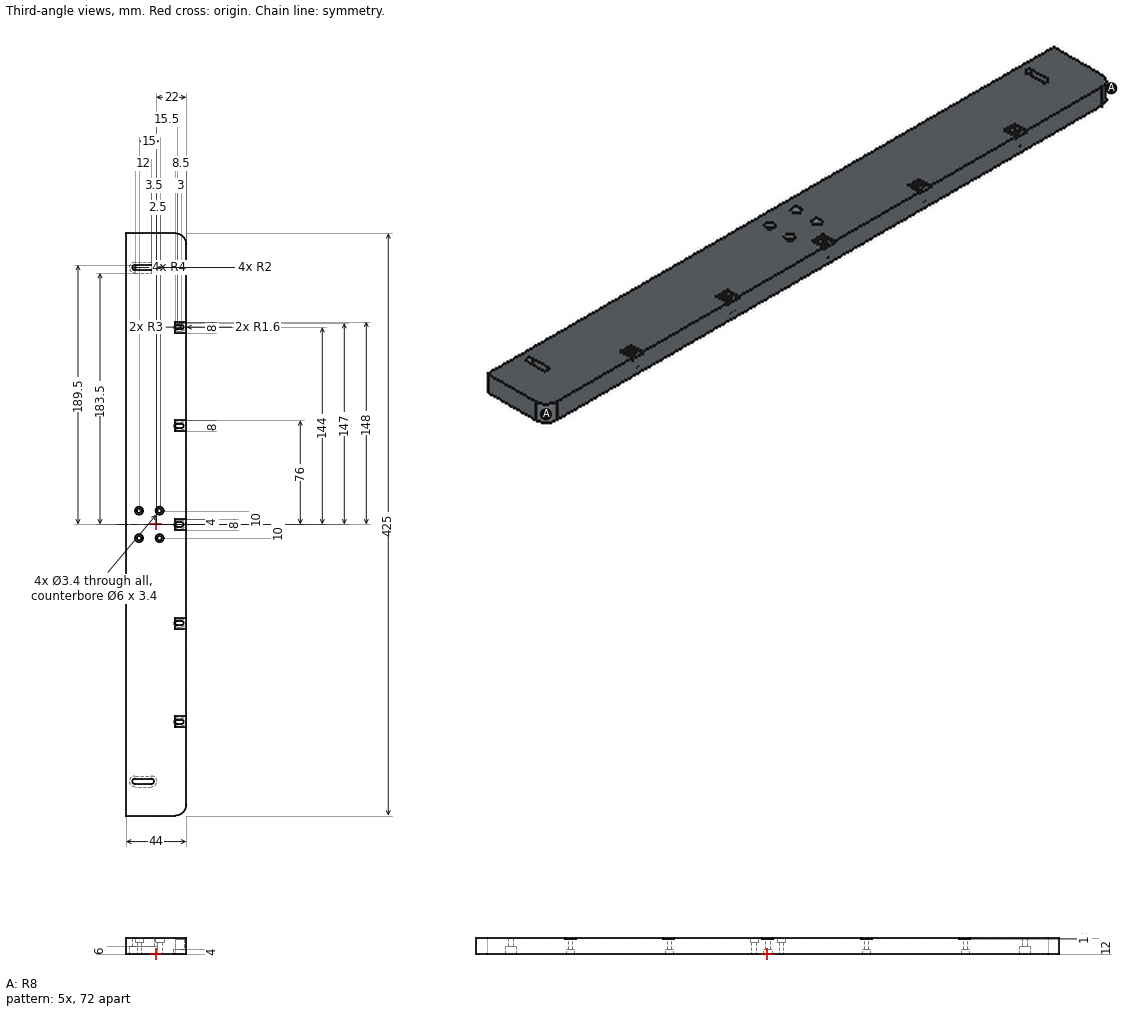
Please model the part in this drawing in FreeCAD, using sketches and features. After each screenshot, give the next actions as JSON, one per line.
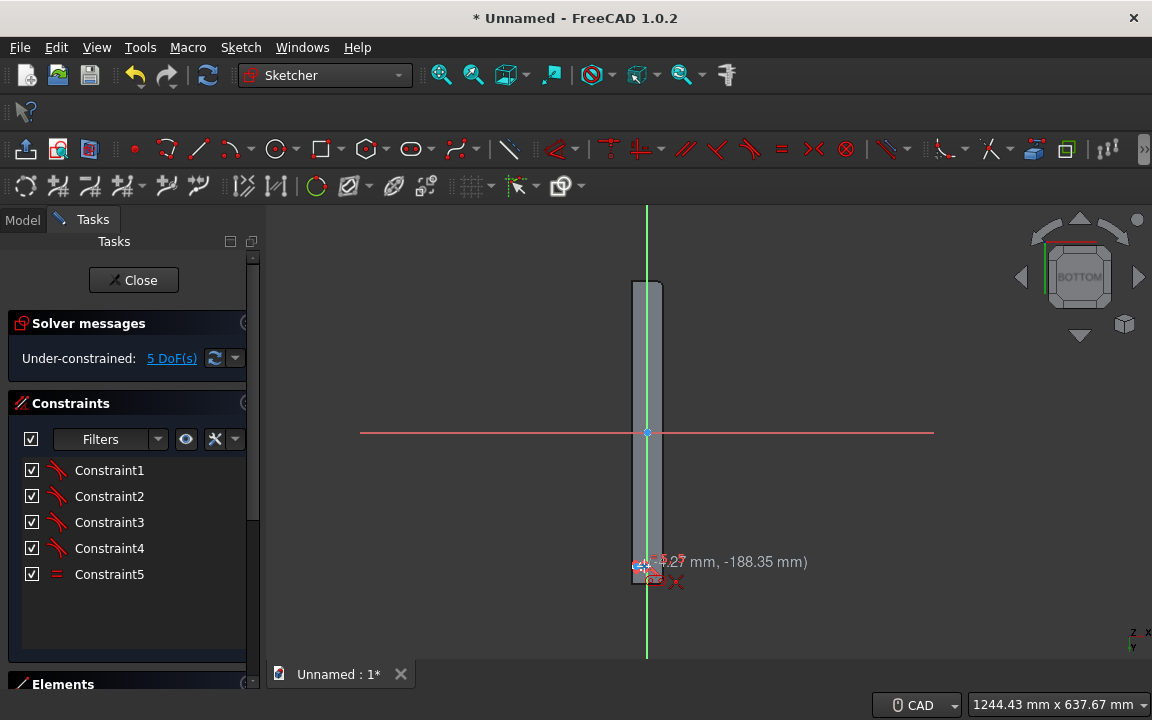
{"action": "scroll", "coordinate": [636, 299], "scroll_direction": "up", "scroll_amount": 11}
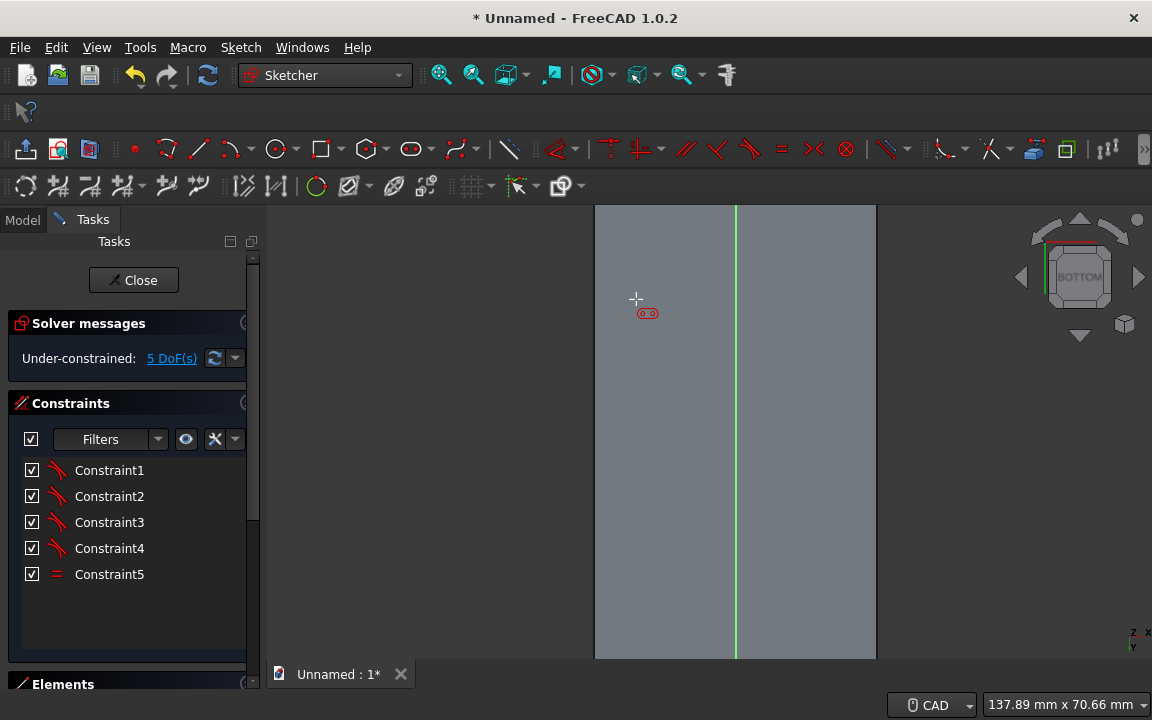
{"action": "scroll", "coordinate": [636, 298], "scroll_direction": "down", "scroll_amount": 11}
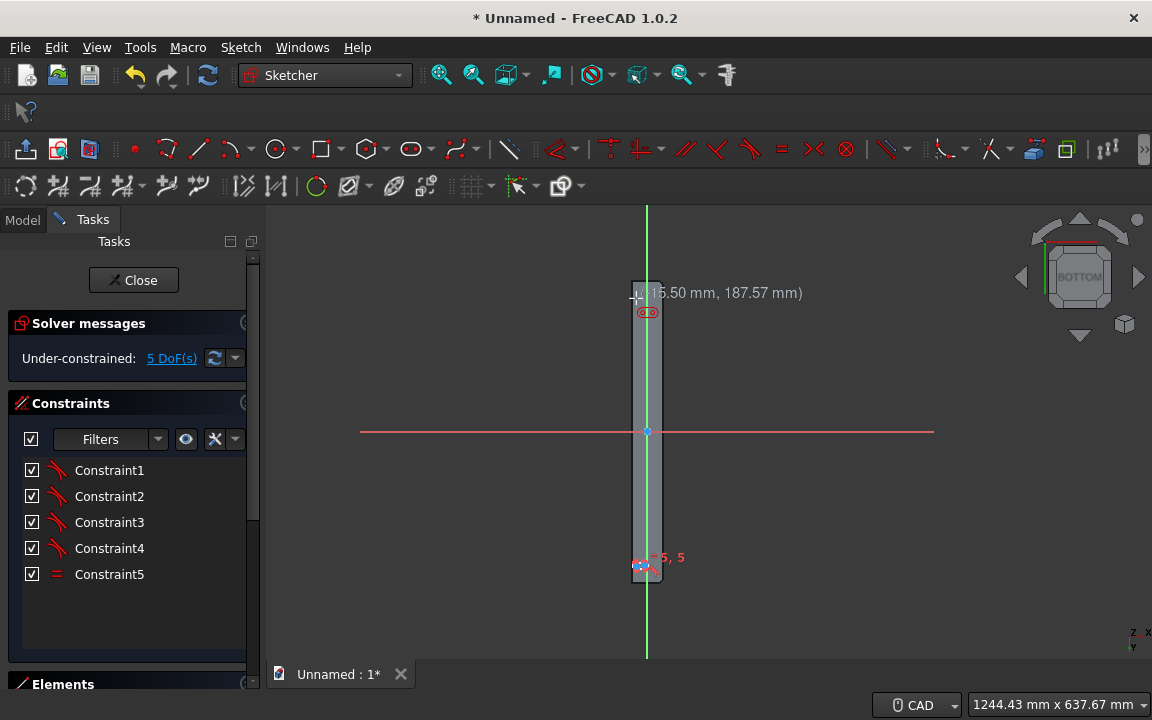
{"action": "scroll", "coordinate": [636, 298], "scroll_direction": "up", "scroll_amount": 2}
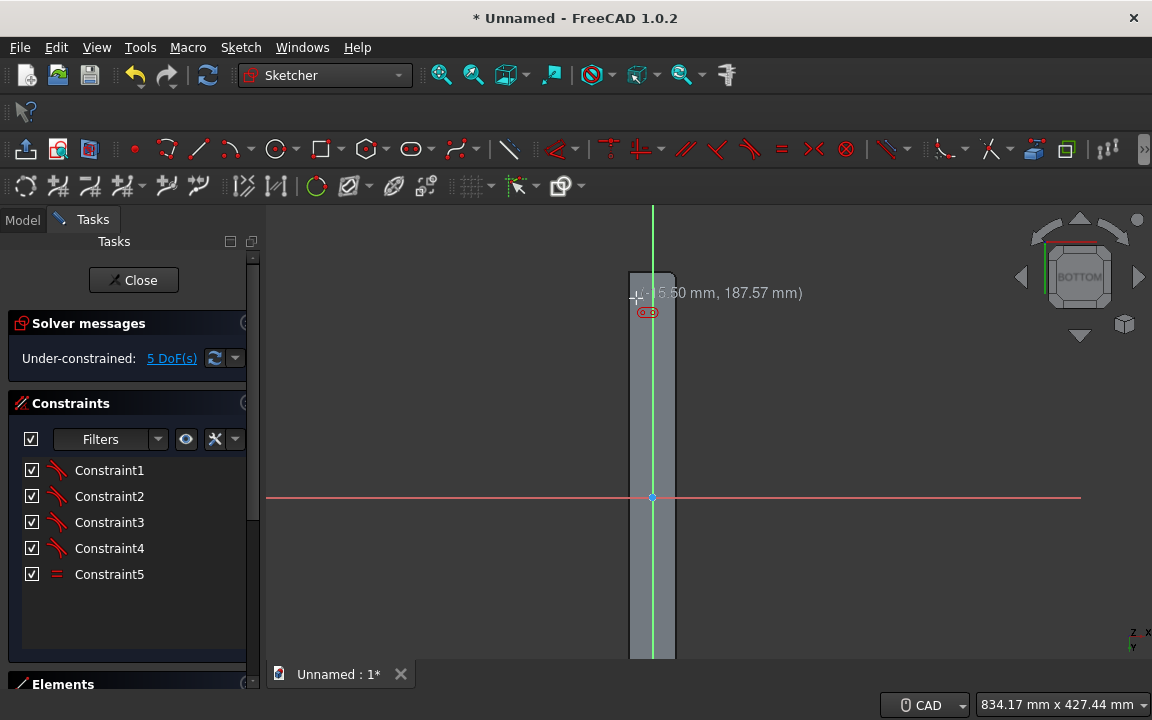
{"action": "left_click", "coordinate": [636, 298]}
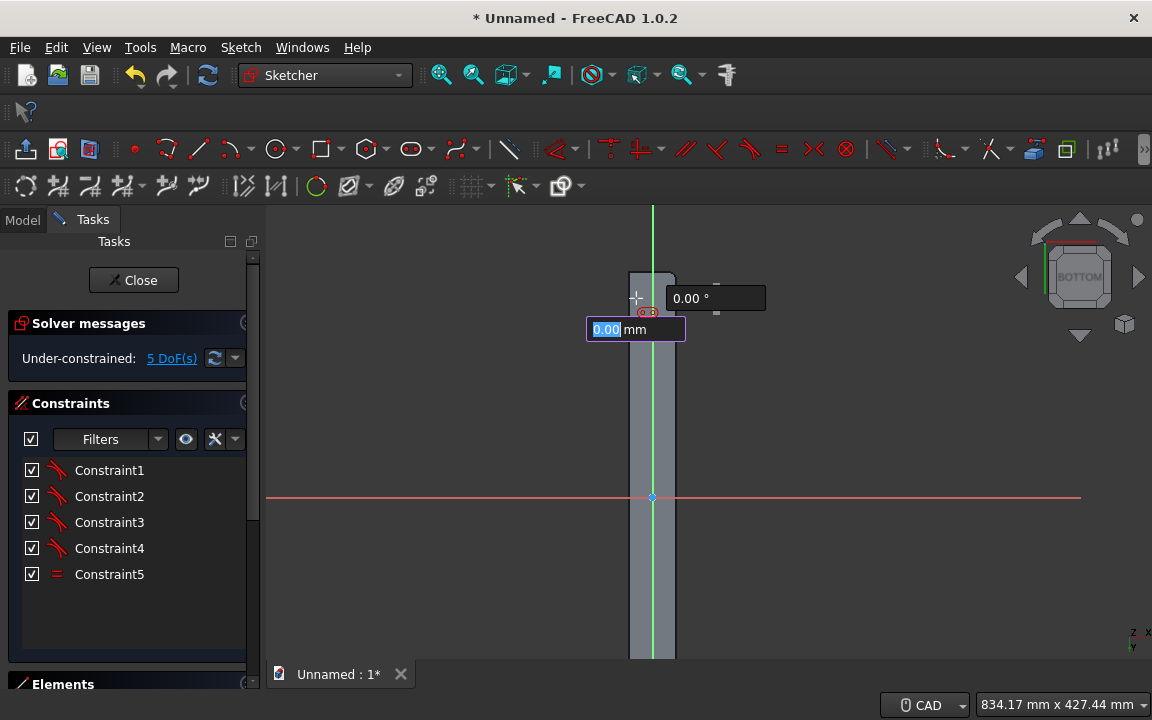
{"action": "scroll", "coordinate": [649, 298], "scroll_direction": "up", "scroll_amount": 8}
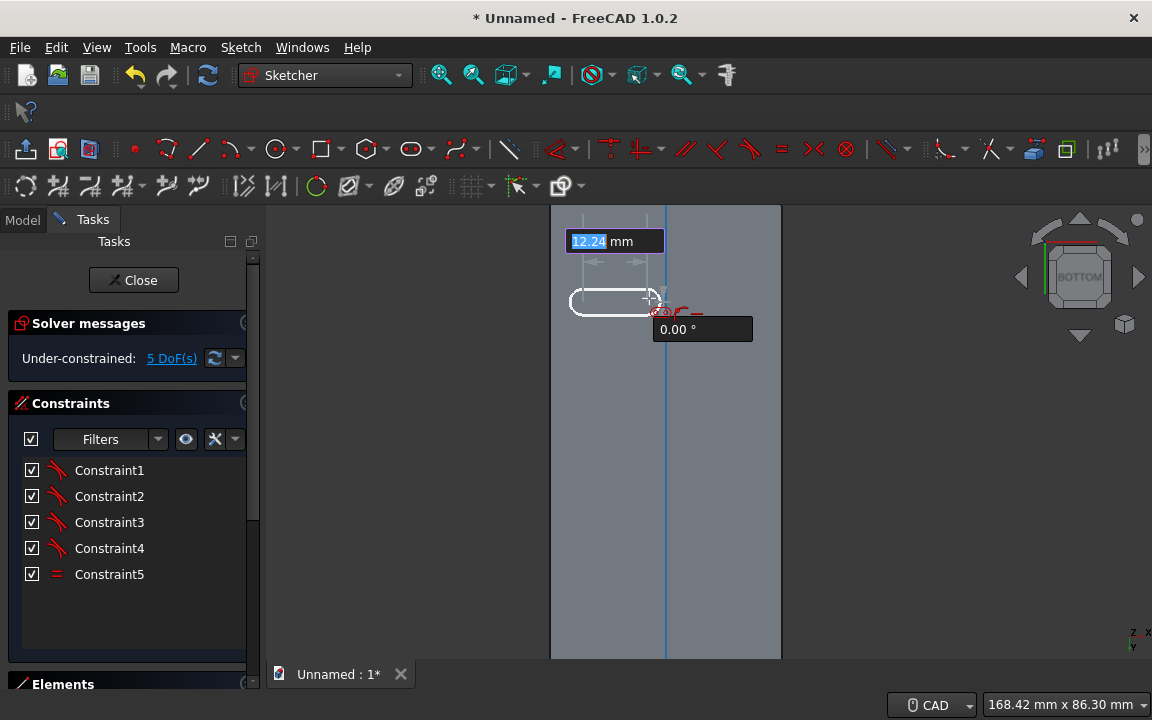
{"action": "left_click", "coordinate": [648, 297]}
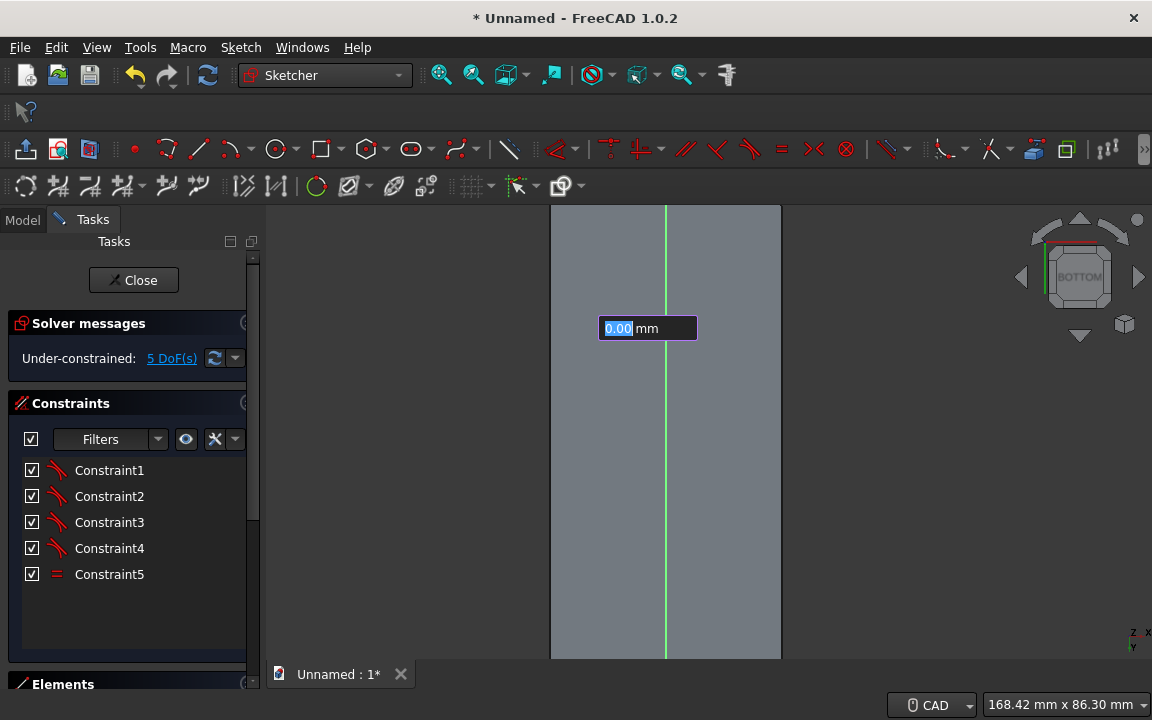
{"action": "left_click", "coordinate": [616, 320]}
{"action": "key", "text": "Escape"}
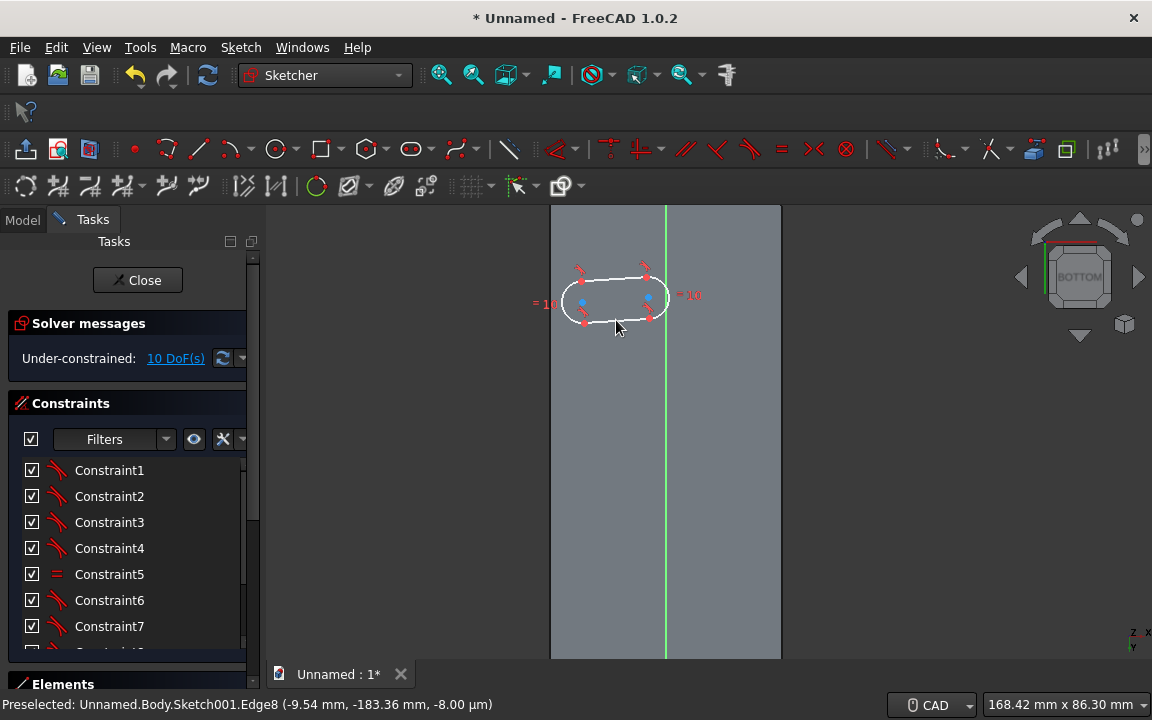
{"action": "scroll", "coordinate": [644, 298], "scroll_direction": "down", "scroll_amount": 10}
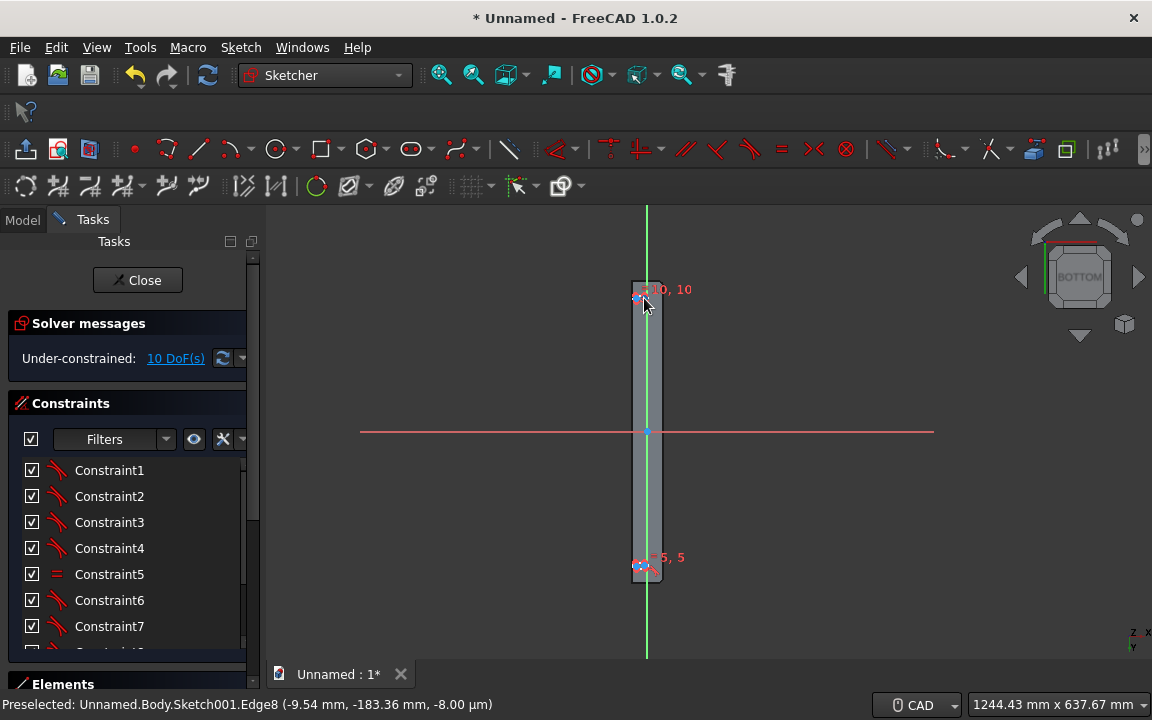
{"action": "scroll", "coordinate": [639, 563], "scroll_direction": "up", "scroll_amount": 9}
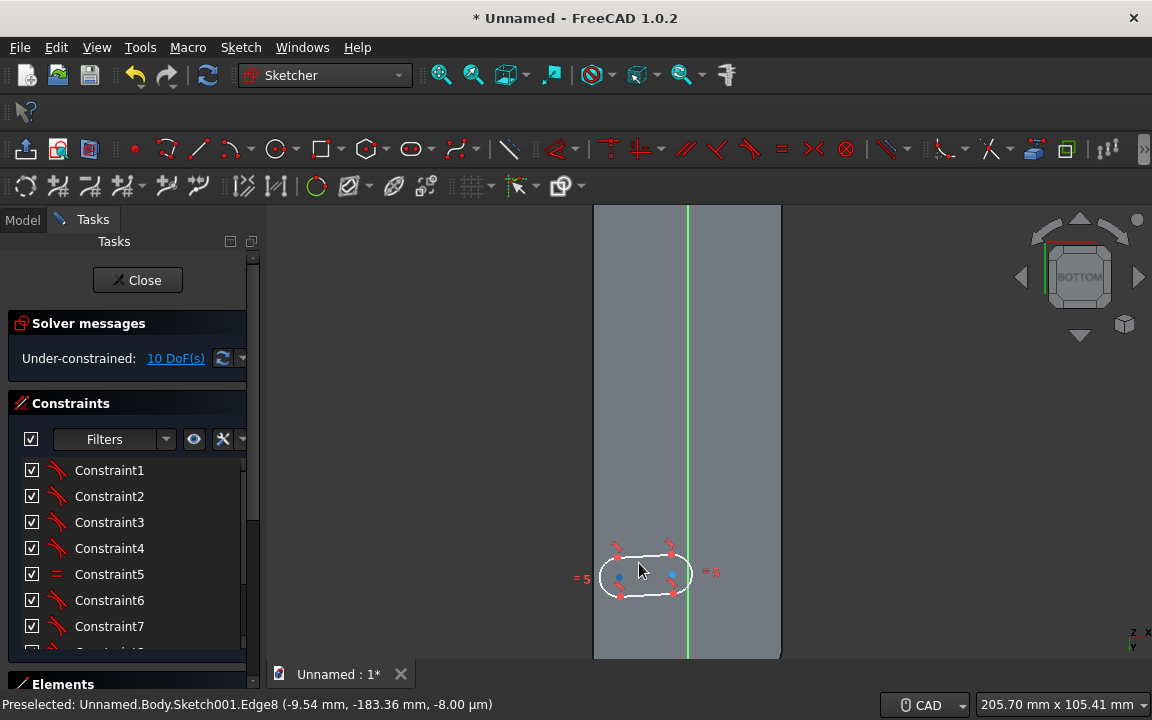
{"action": "left_click", "coordinate": [634, 557]}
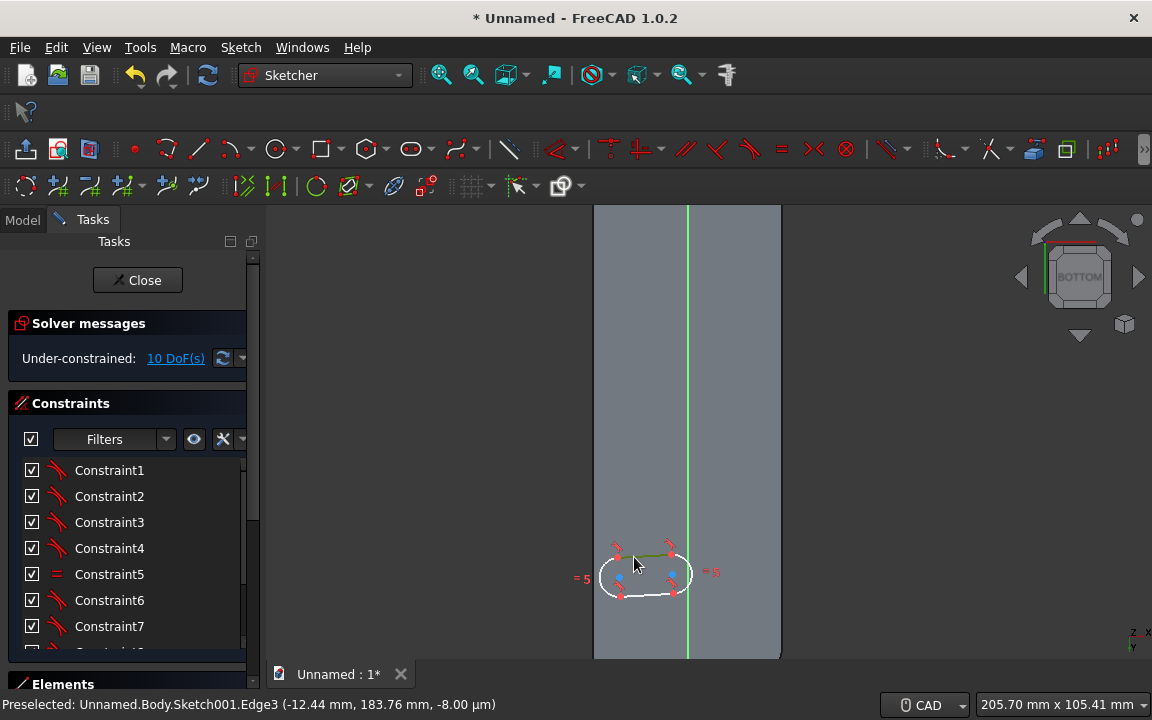
{"action": "left_click", "coordinate": [664, 150]}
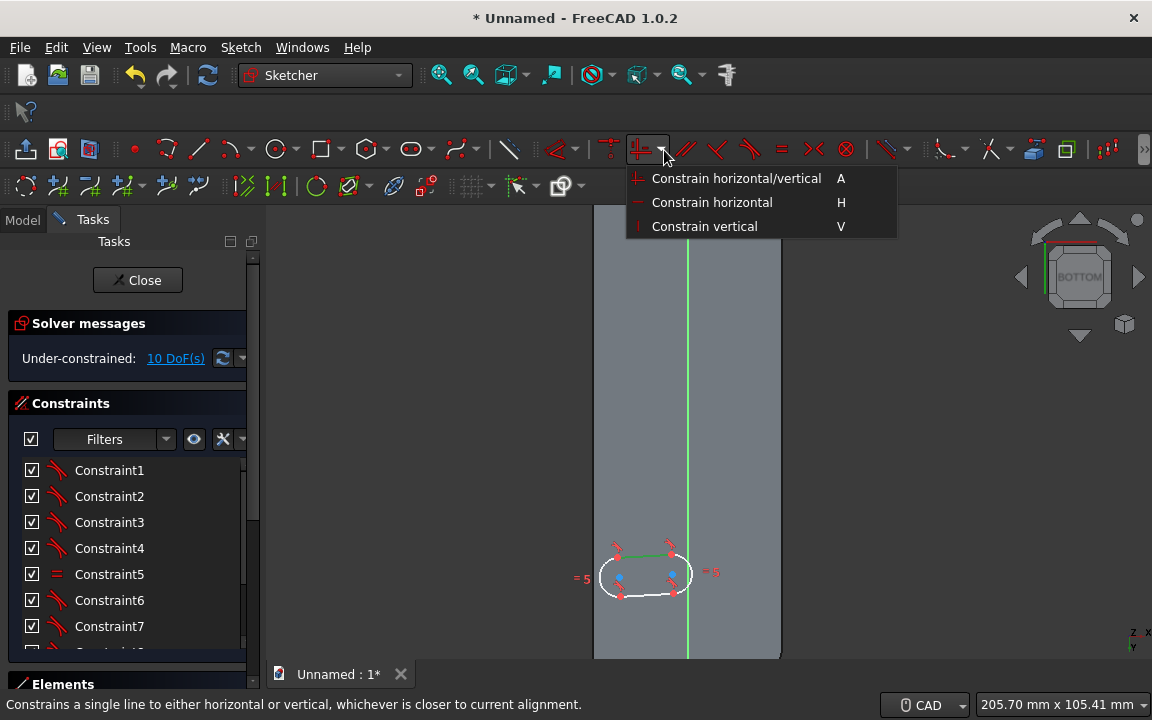
{"action": "left_click", "coordinate": [762, 202]}